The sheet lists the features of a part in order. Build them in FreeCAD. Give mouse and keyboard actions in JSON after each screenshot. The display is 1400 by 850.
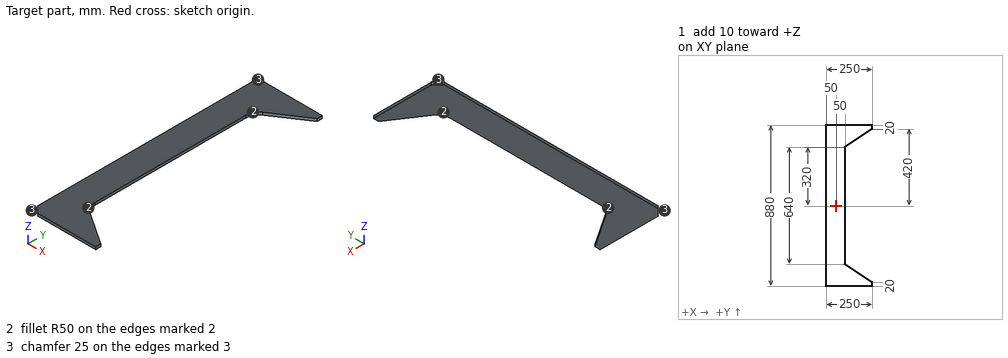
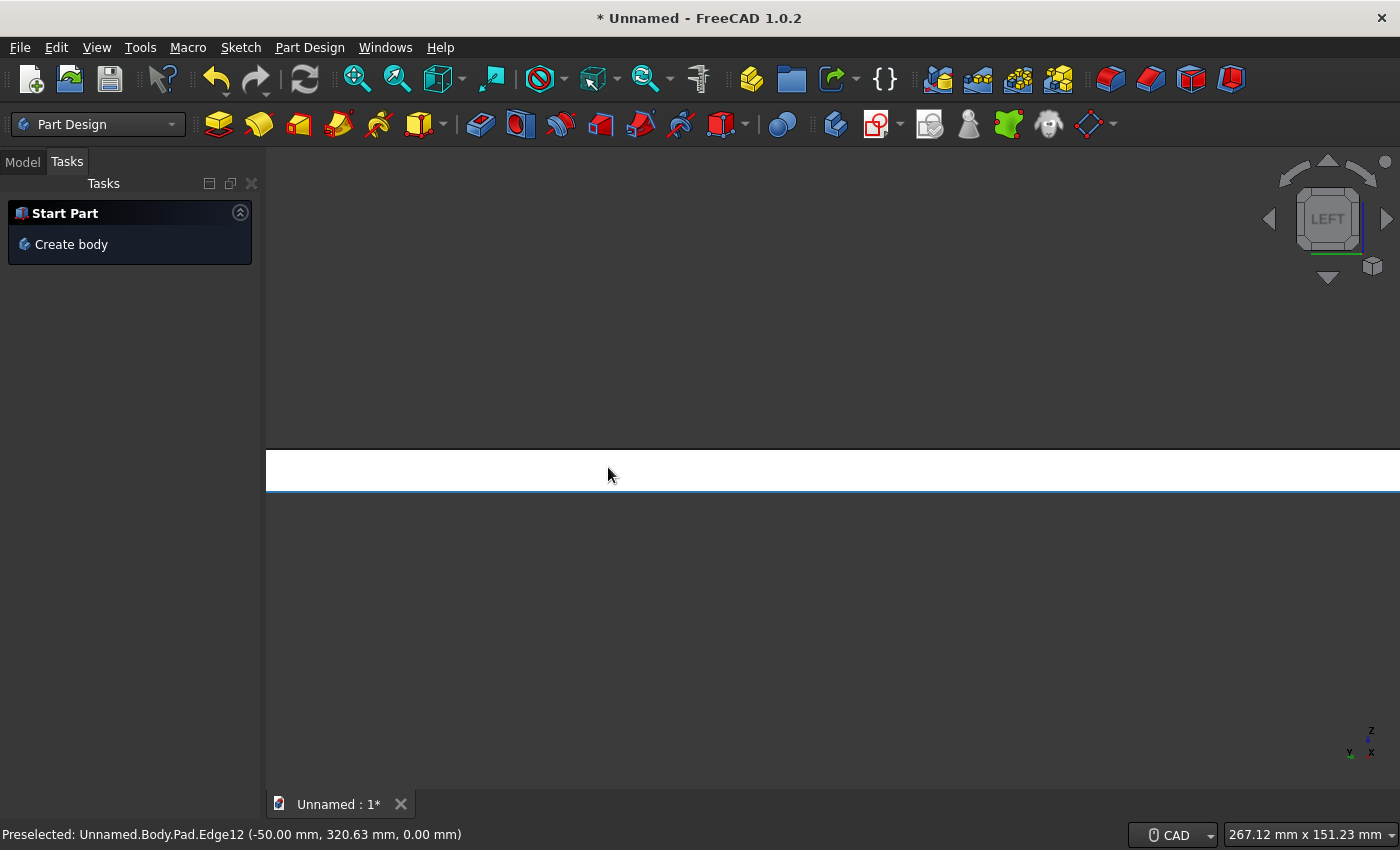
{"action": "left_click", "coordinate": [358, 80]}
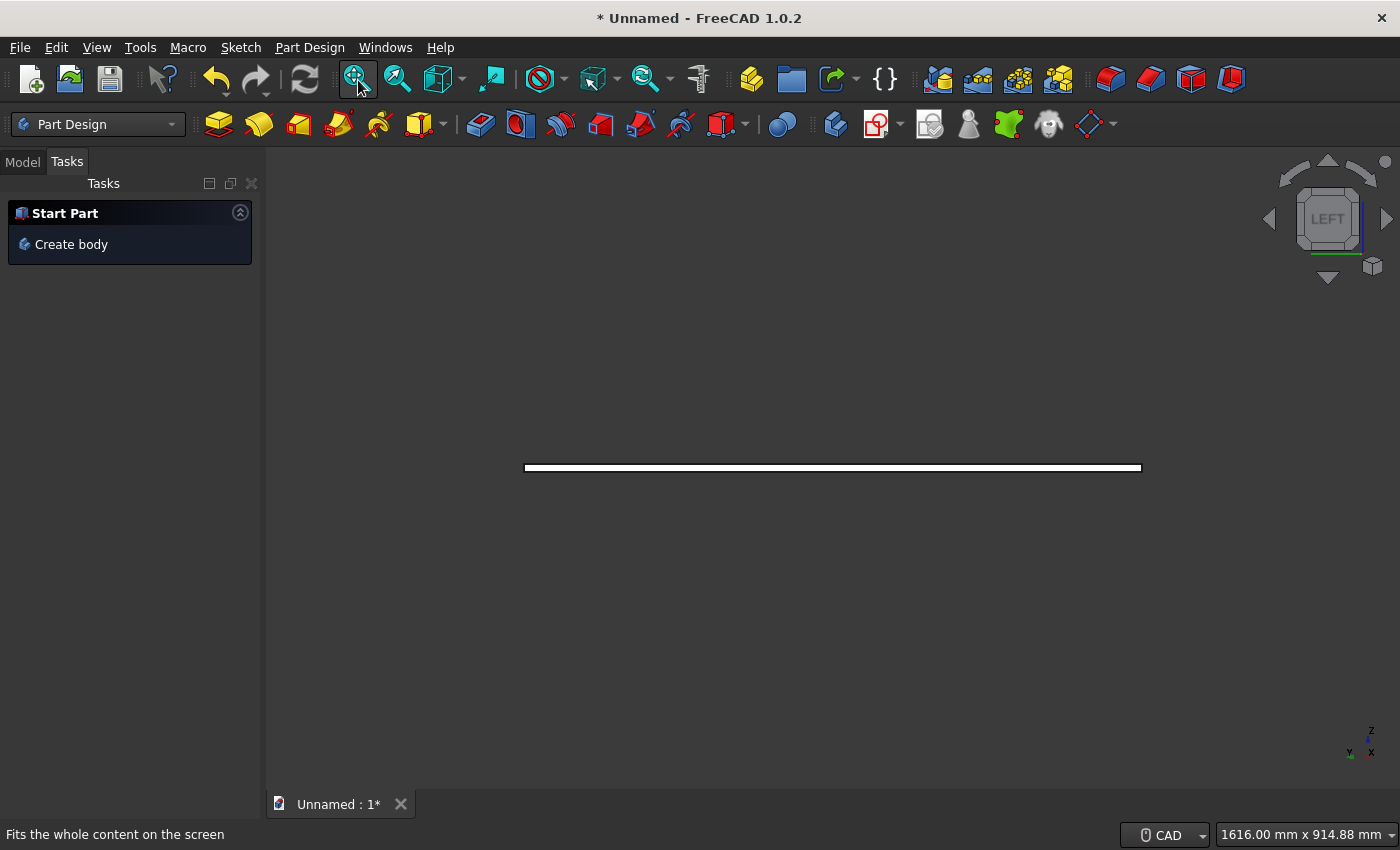
{"action": "key", "text": "v 3"}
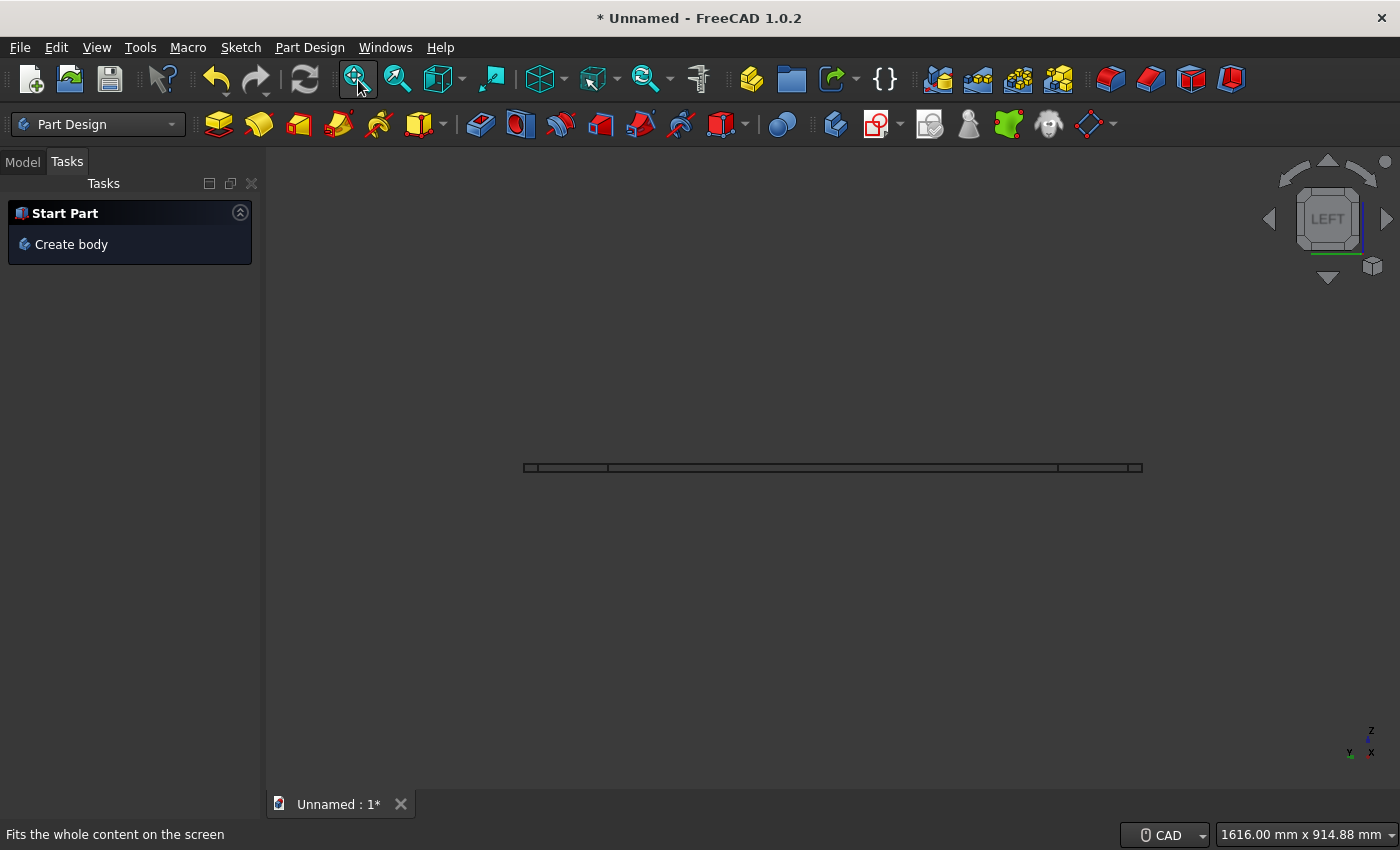
{"action": "key", "text": "0"}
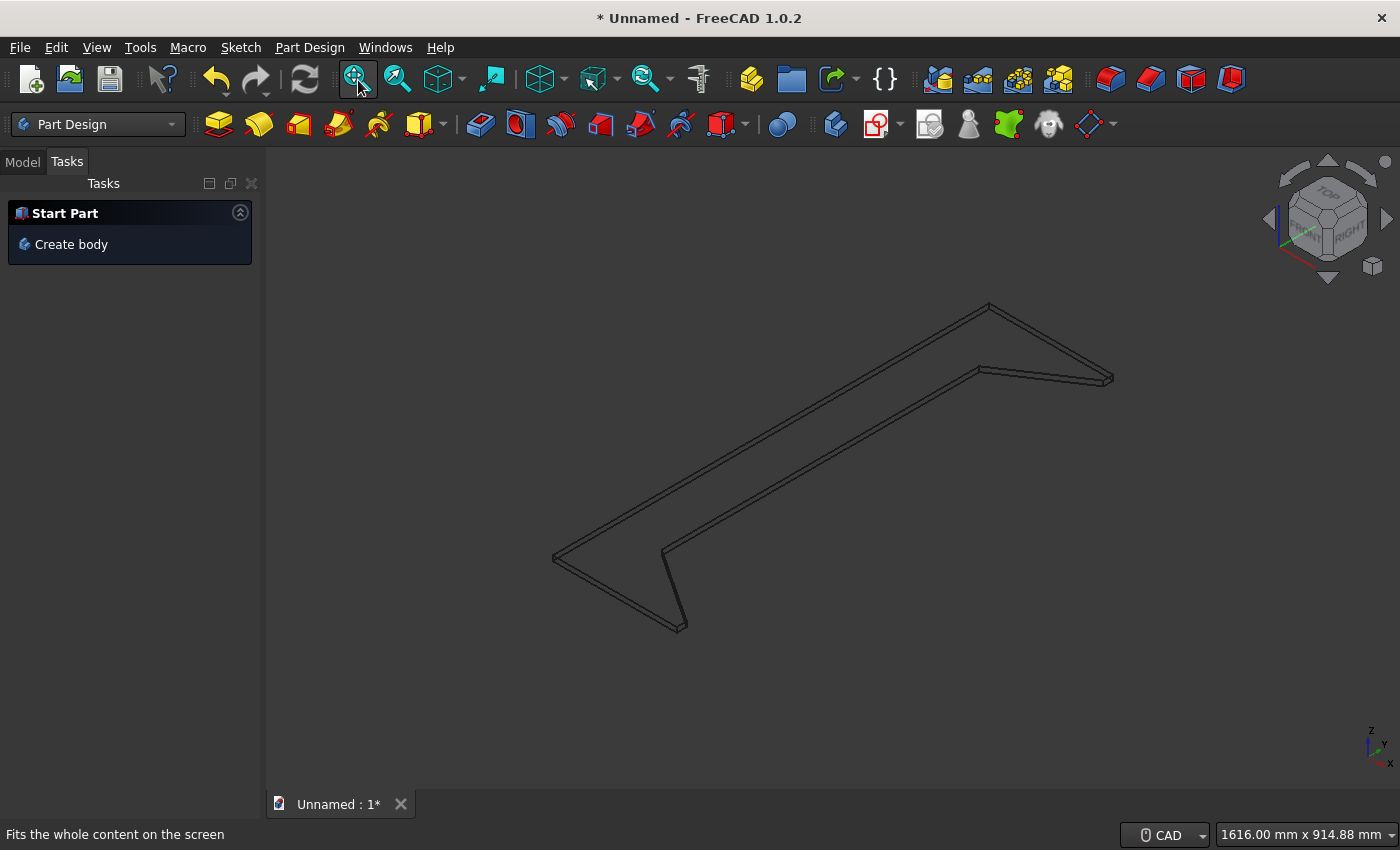
{"action": "scroll", "coordinate": [979, 368], "scroll_direction": "up", "scroll_amount": 9}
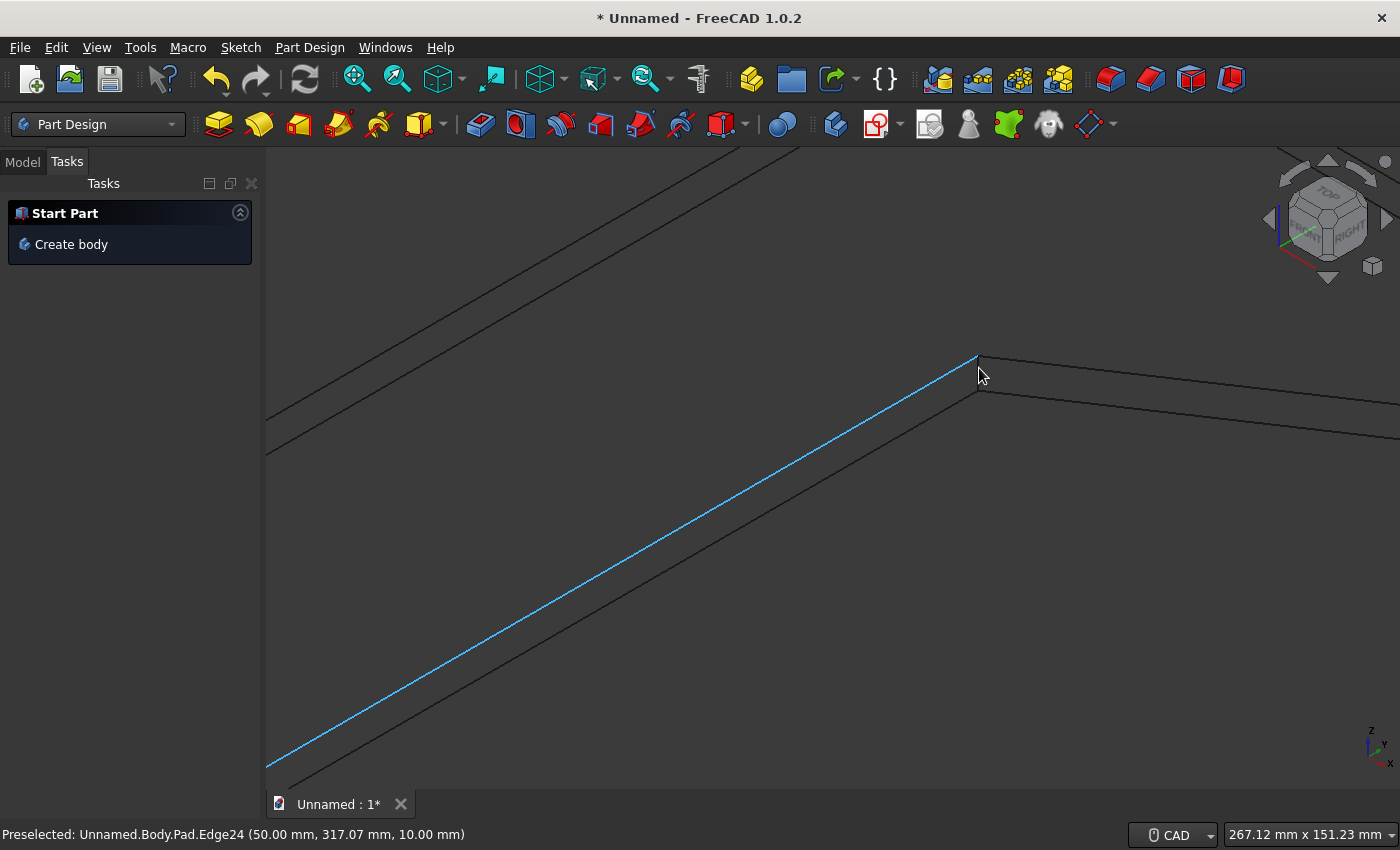
{"action": "left_click", "coordinate": [978, 372]}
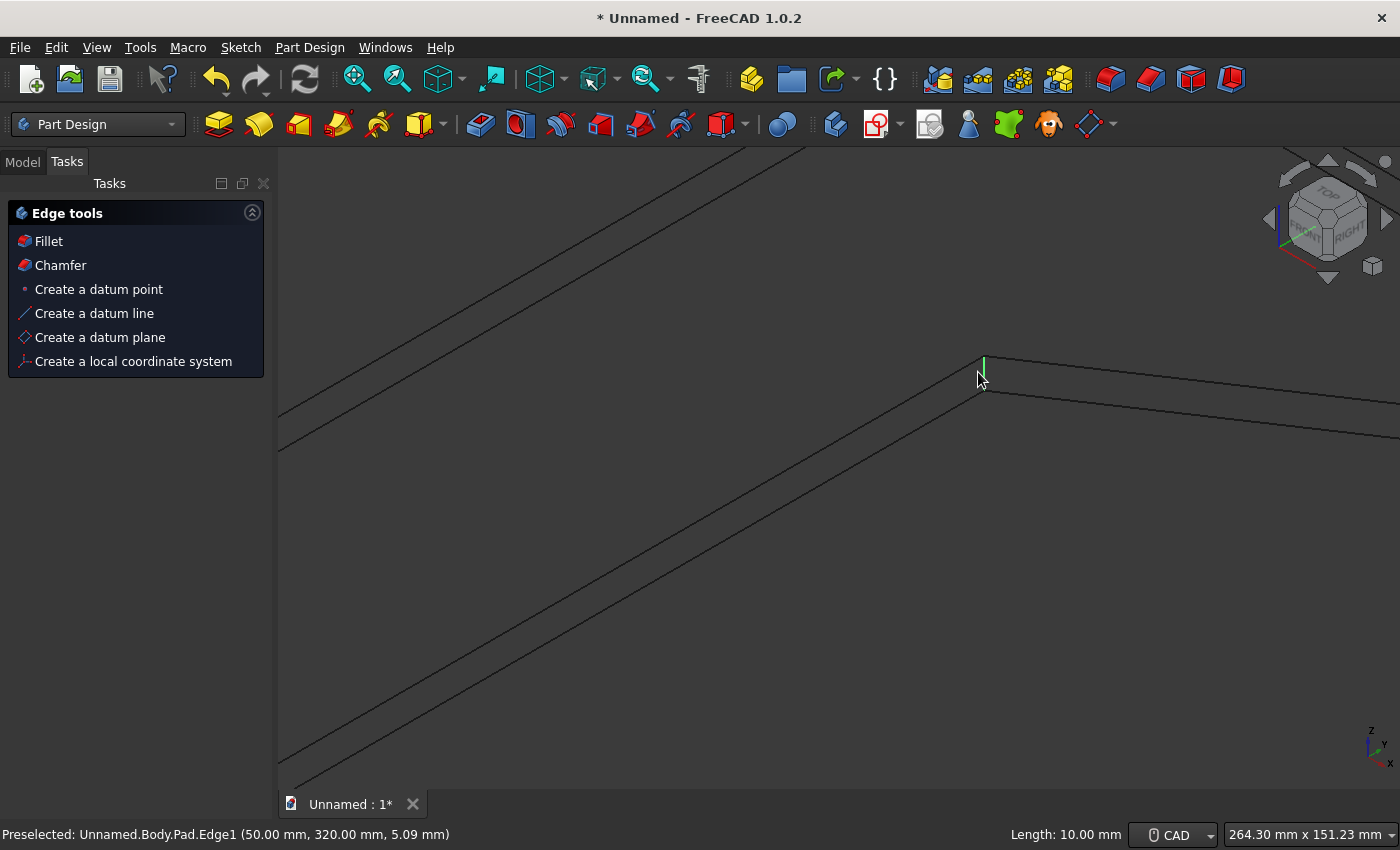
{"action": "key", "text": "v f"}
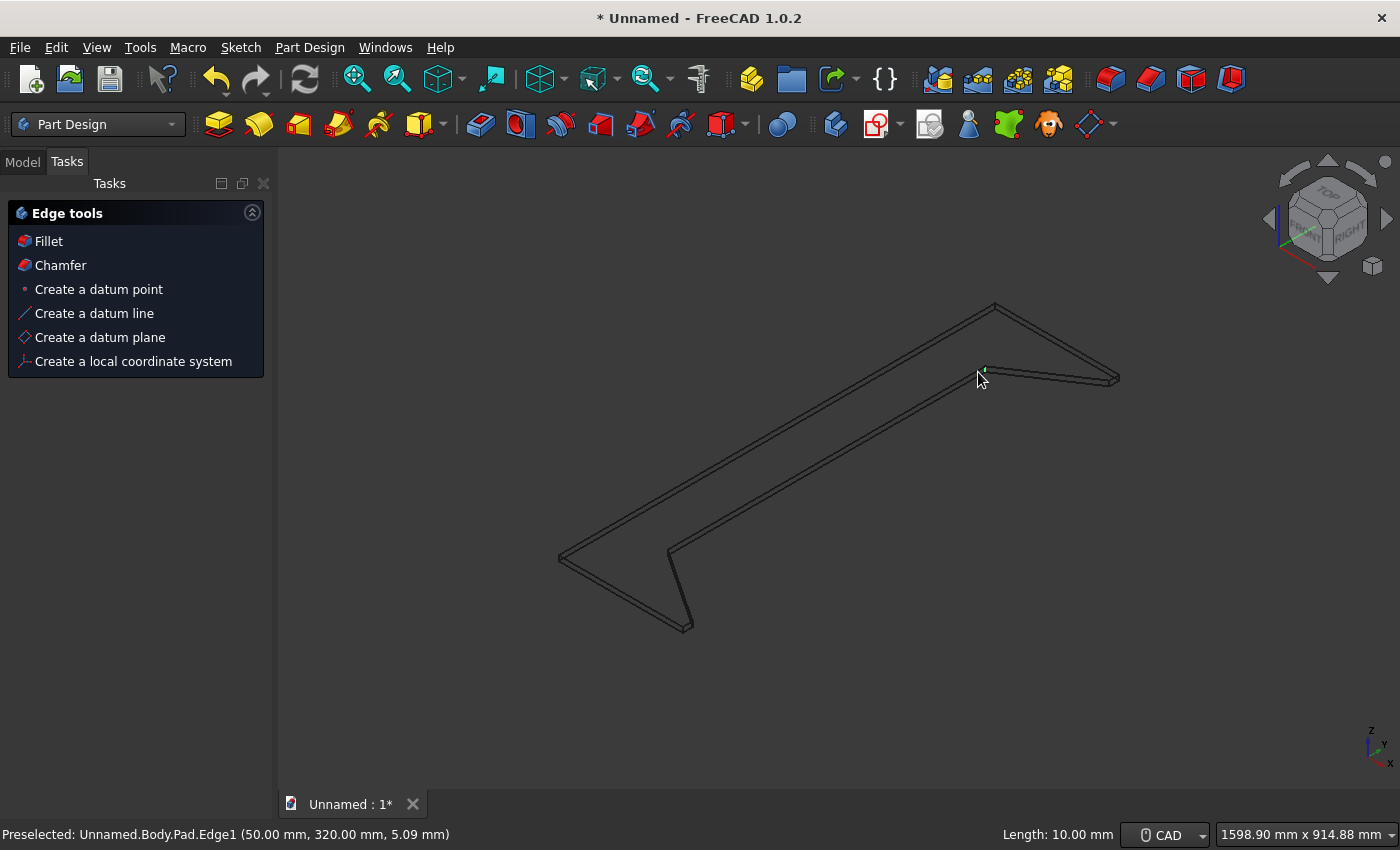
{"action": "key", "text": "2"}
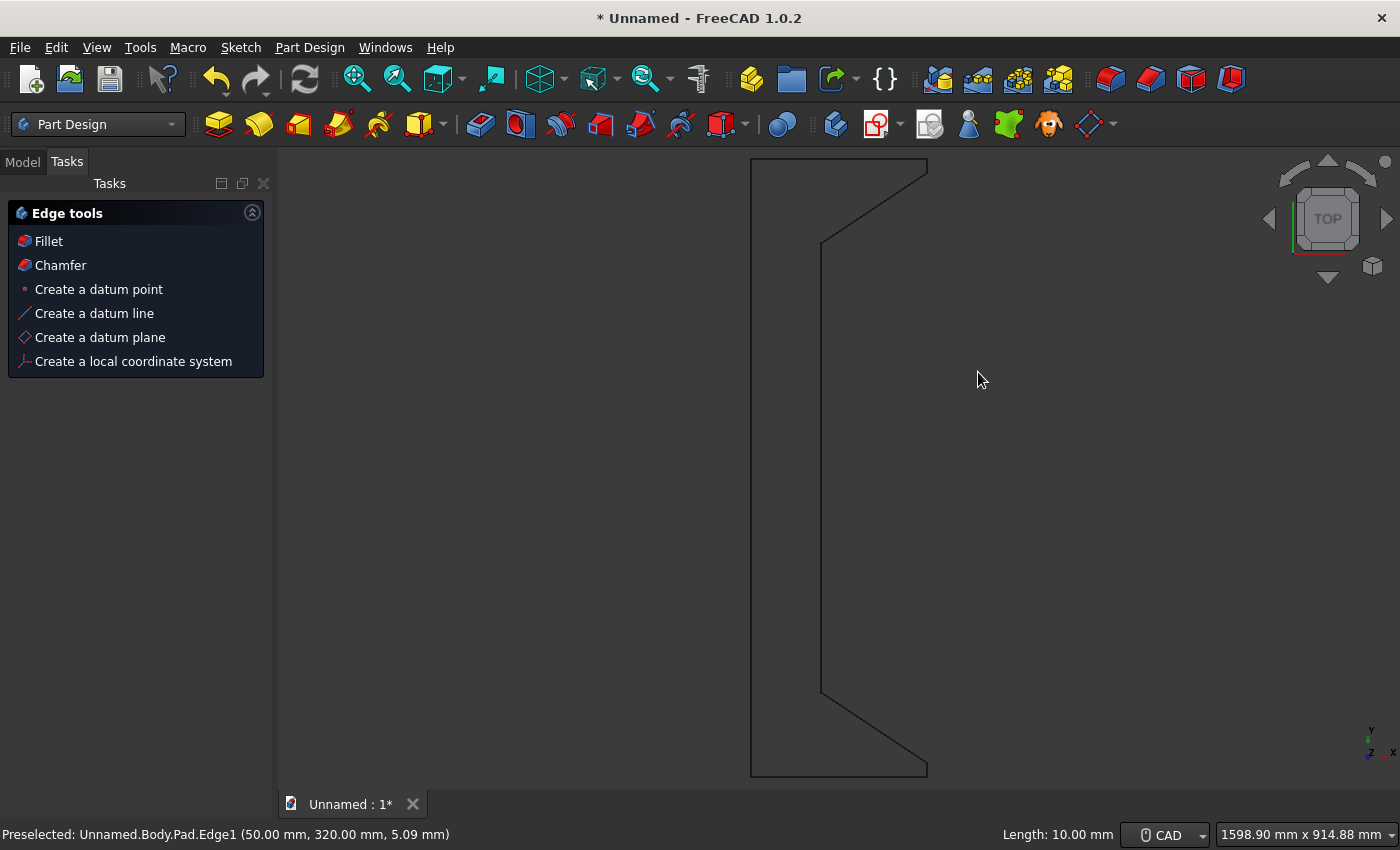
{"action": "scroll", "coordinate": [821, 692], "scroll_direction": "up", "scroll_amount": 9}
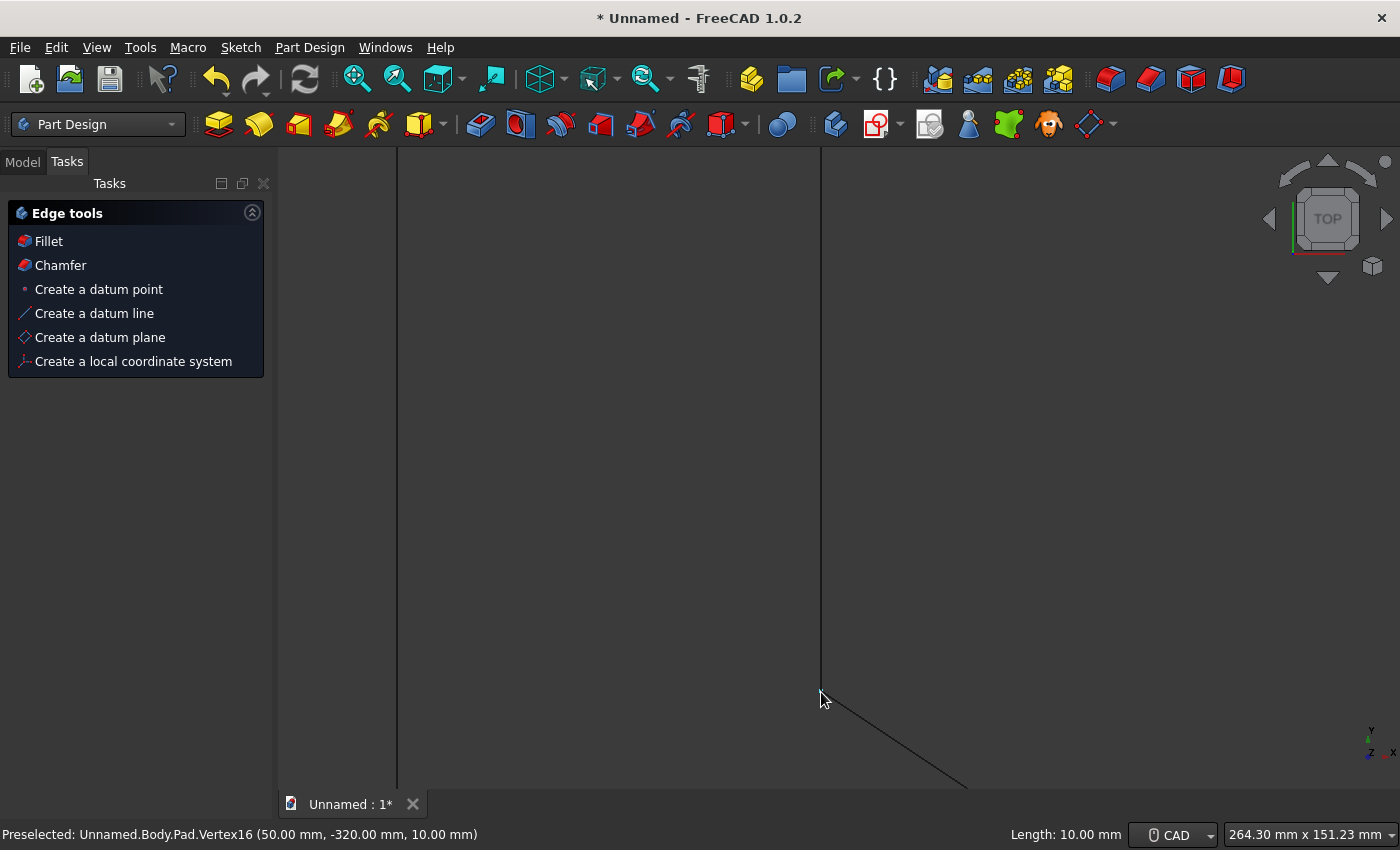
{"action": "key", "text": "v f"}